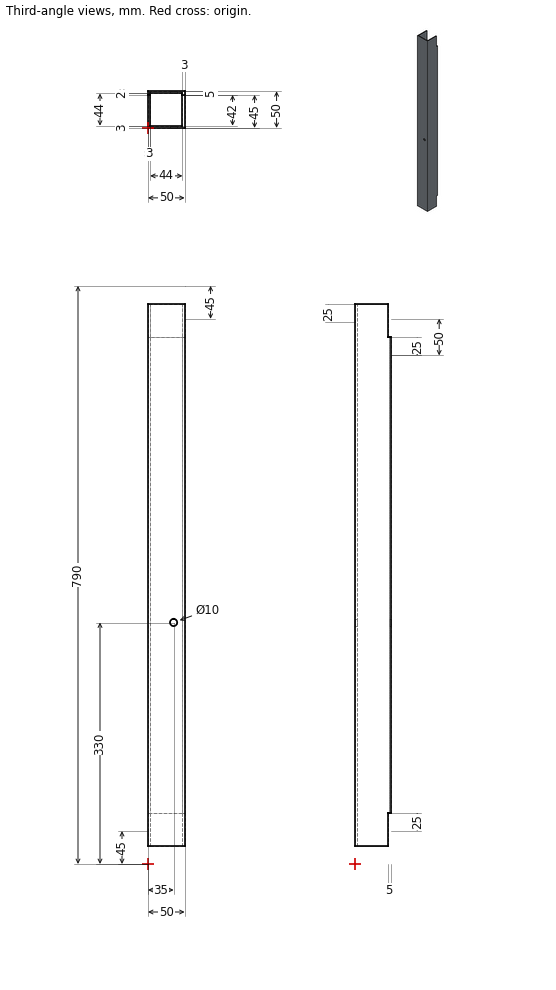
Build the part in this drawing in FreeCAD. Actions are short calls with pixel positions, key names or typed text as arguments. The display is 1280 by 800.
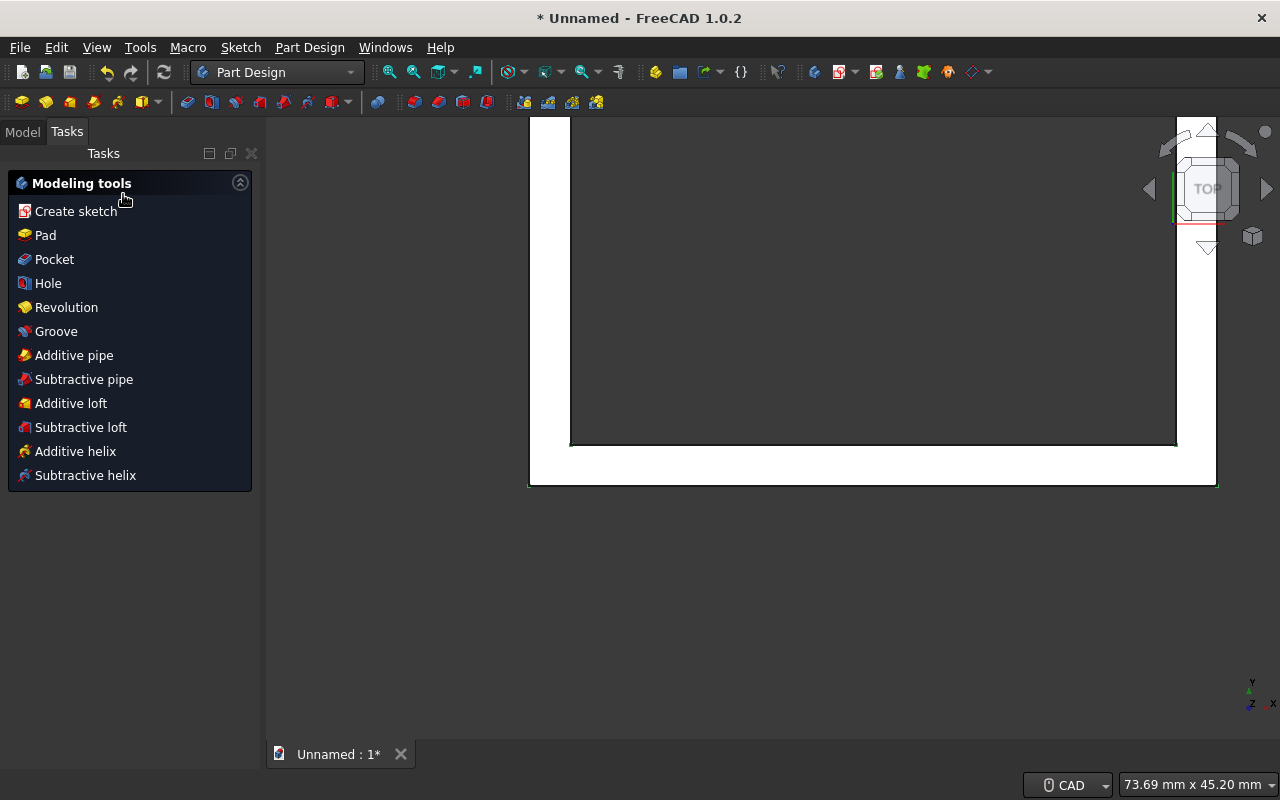
click(22, 102)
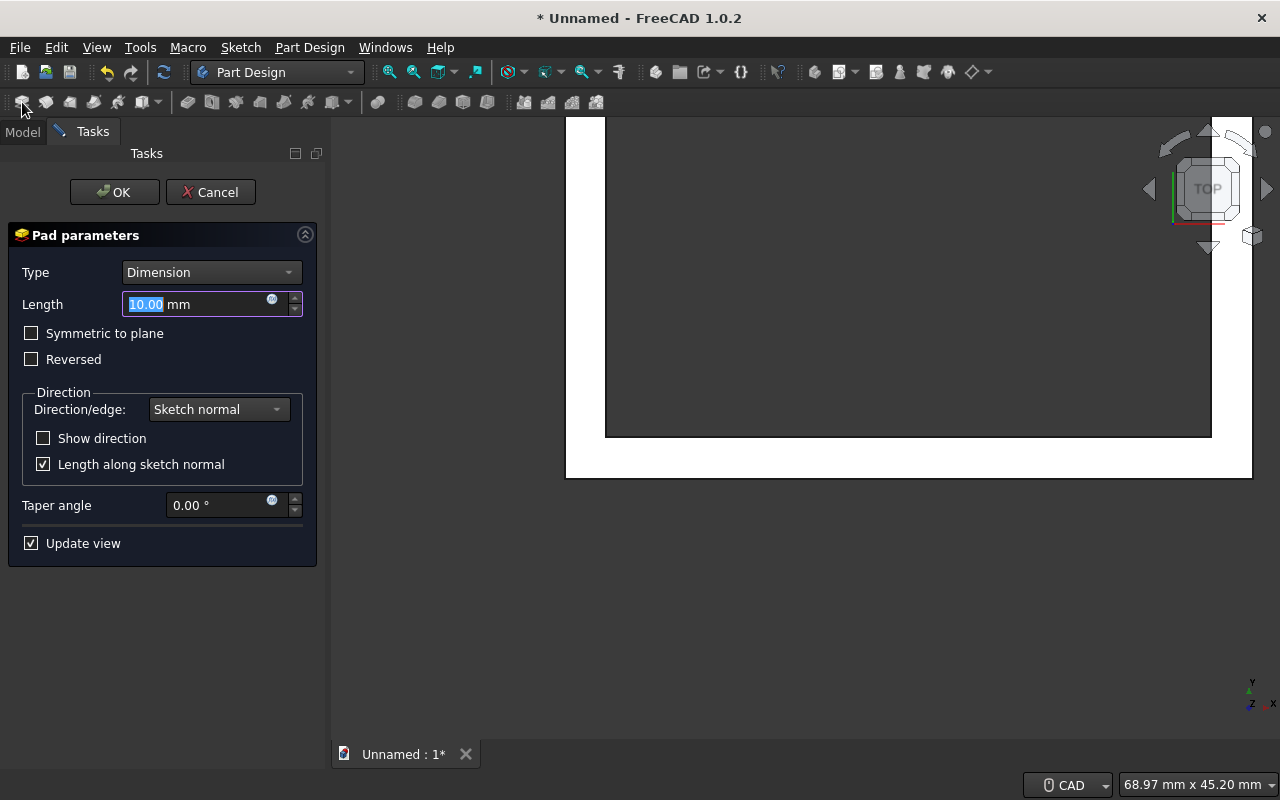
text(25)
key(Tab)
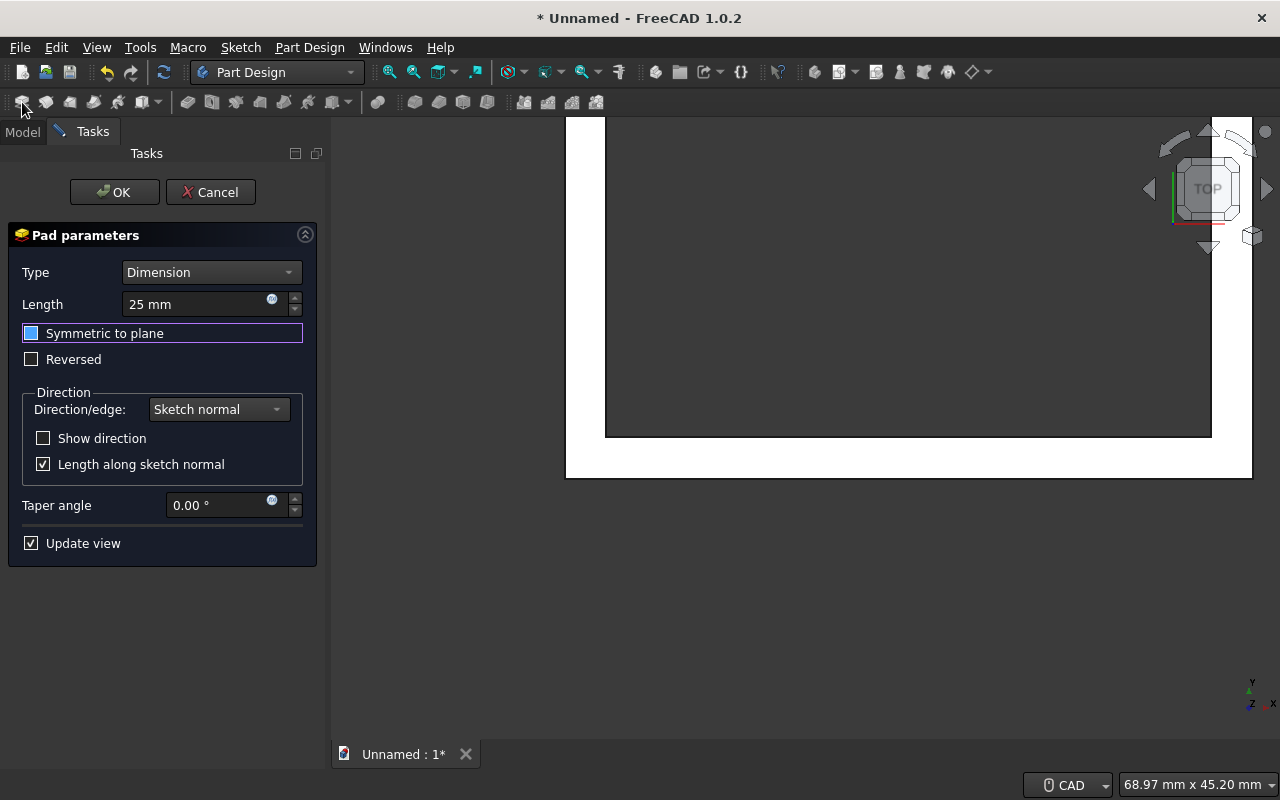
click(115, 192)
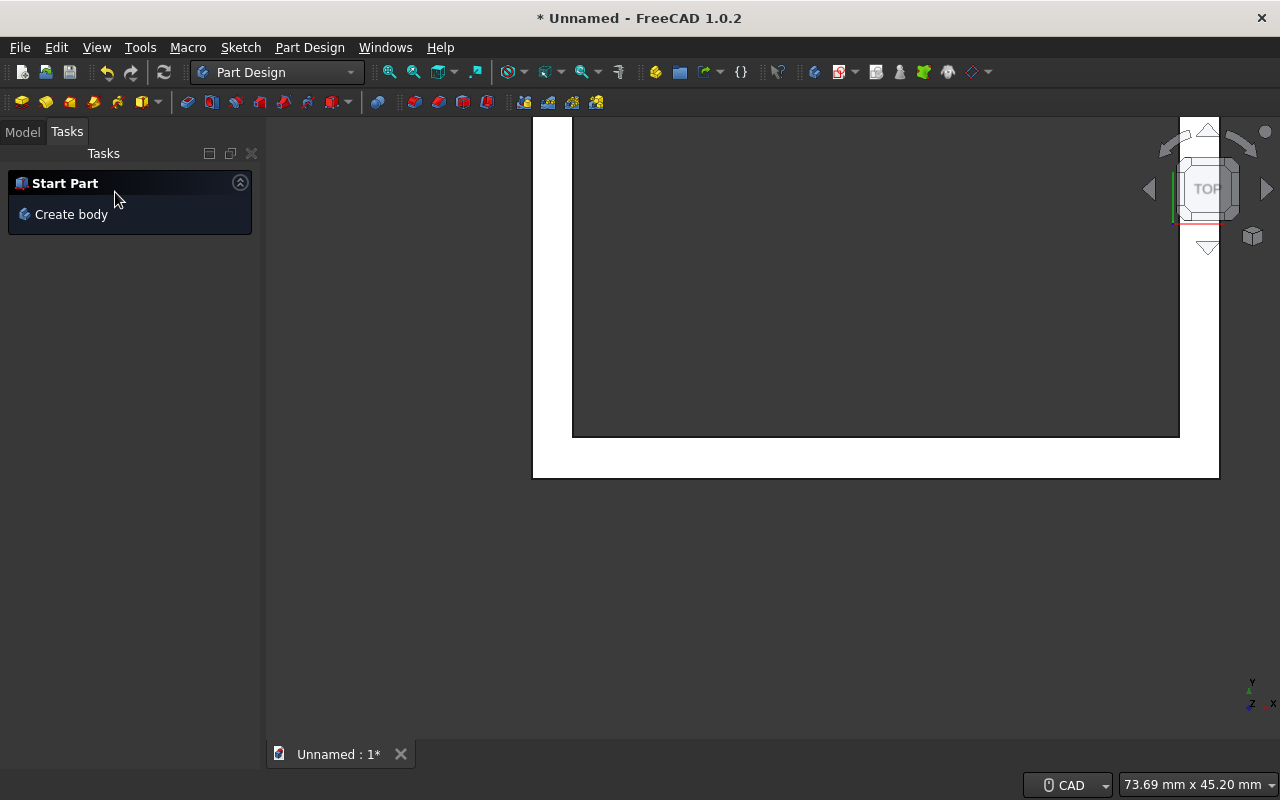
click(390, 72)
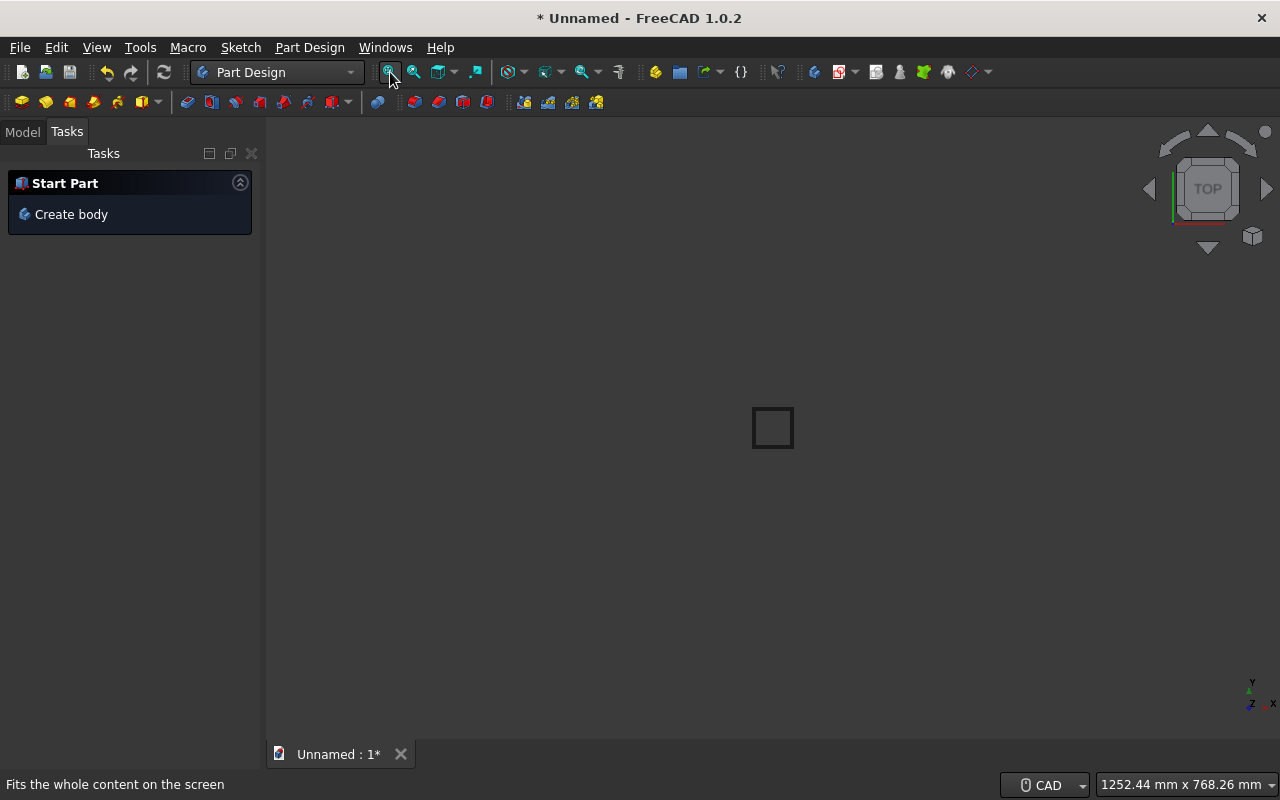
click(840, 72)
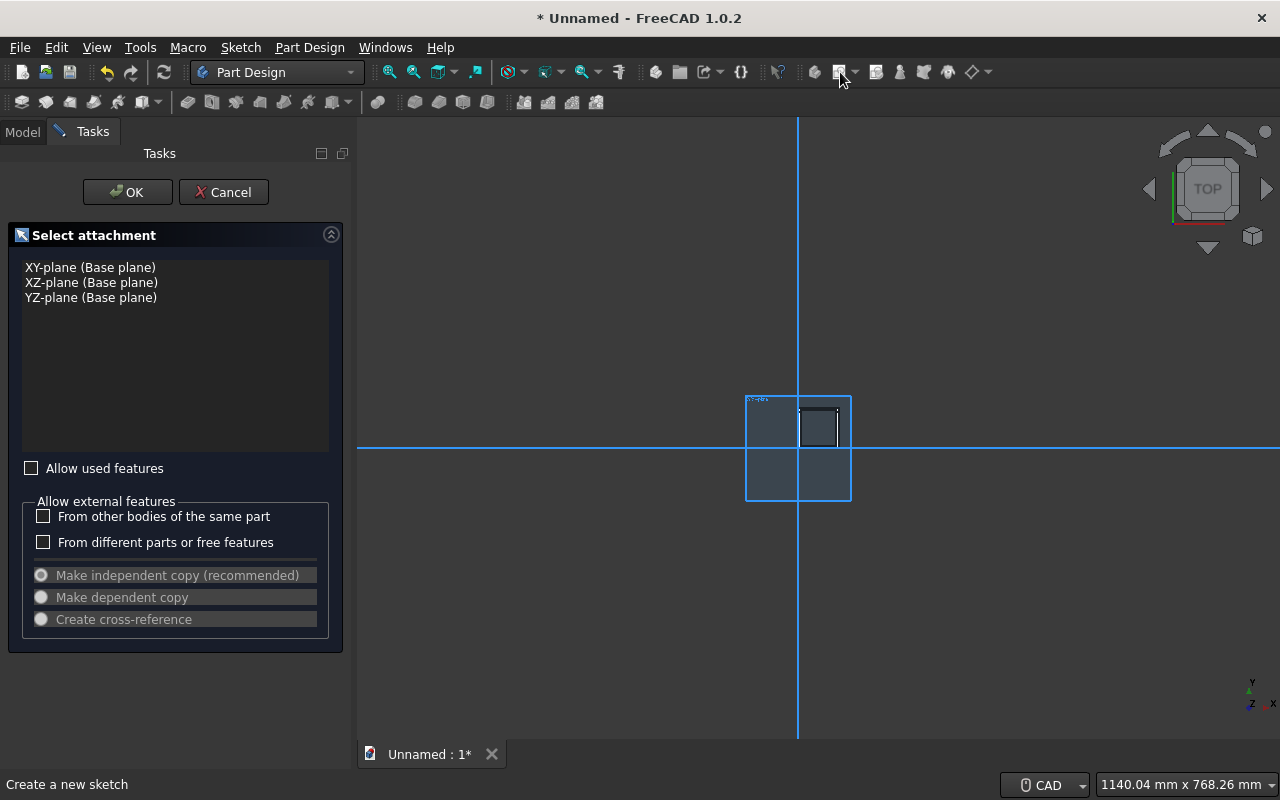
click(82, 268)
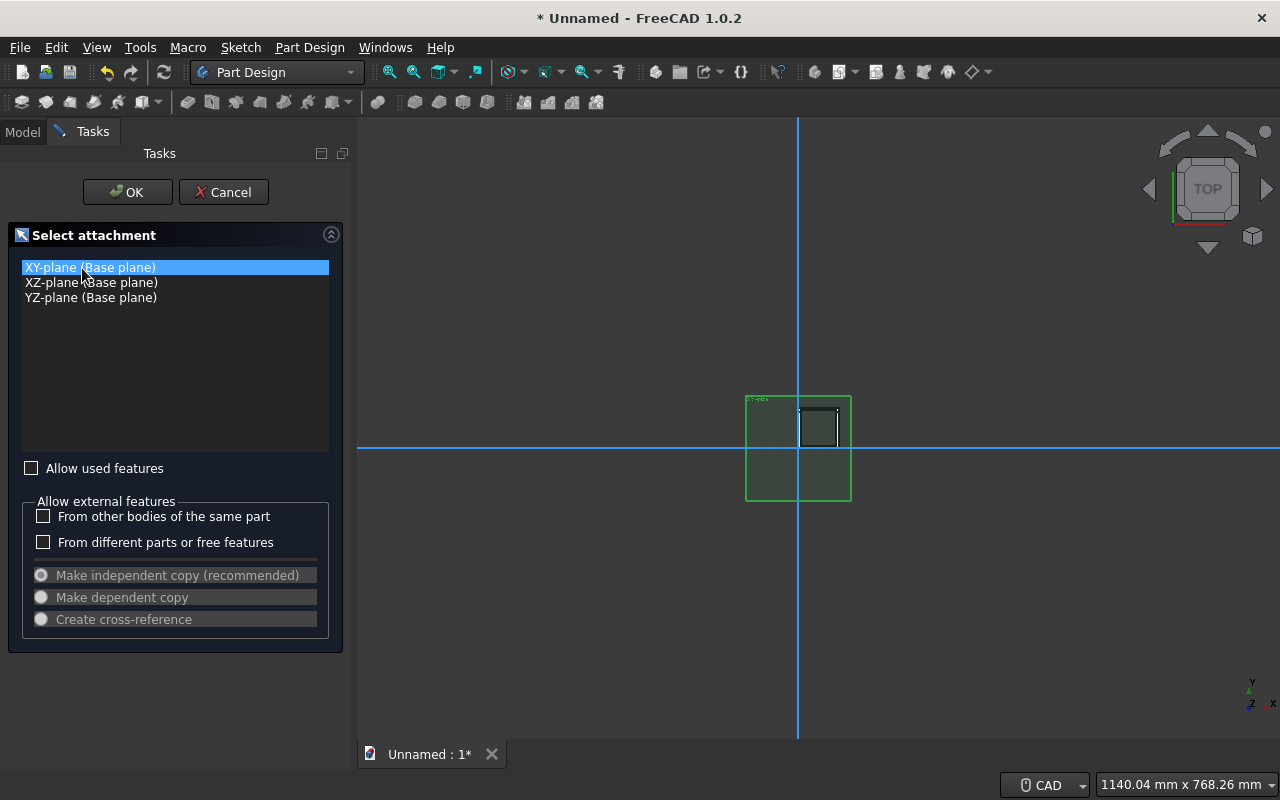
click(128, 192)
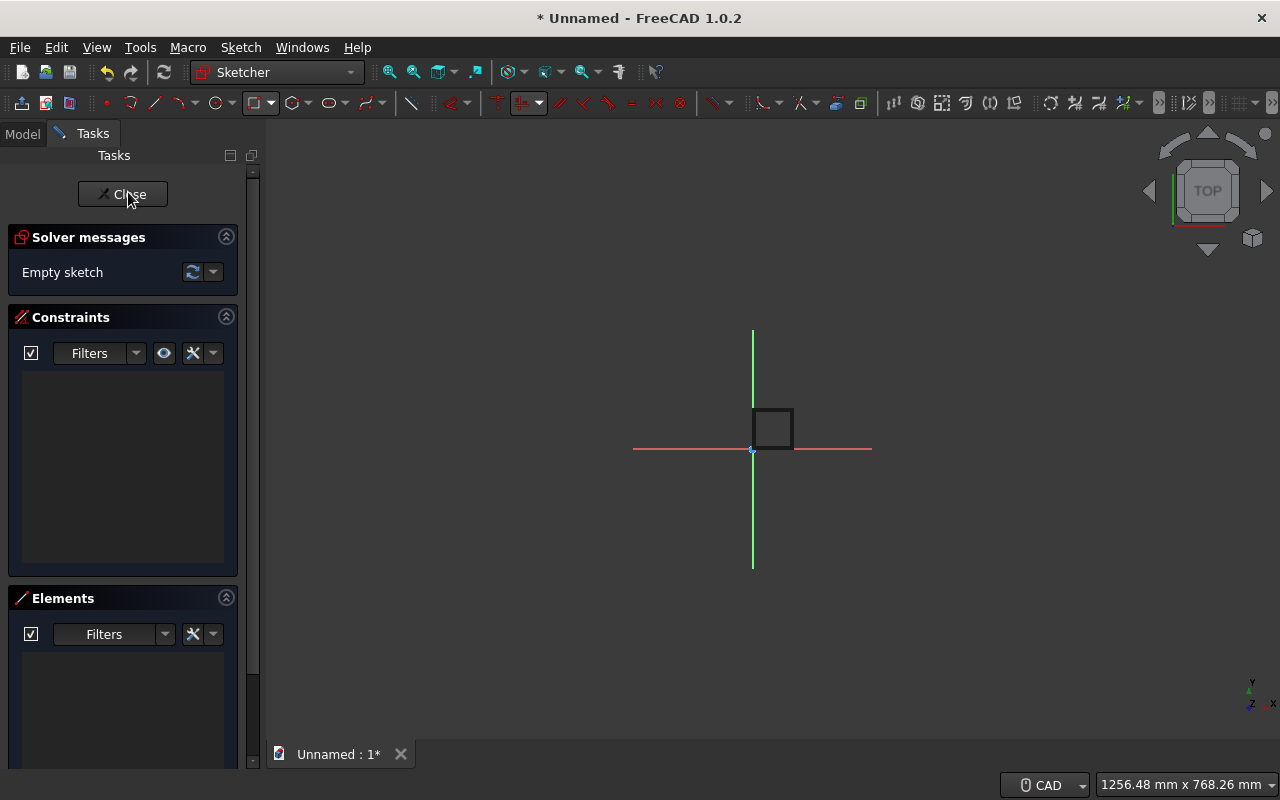
click(70, 104)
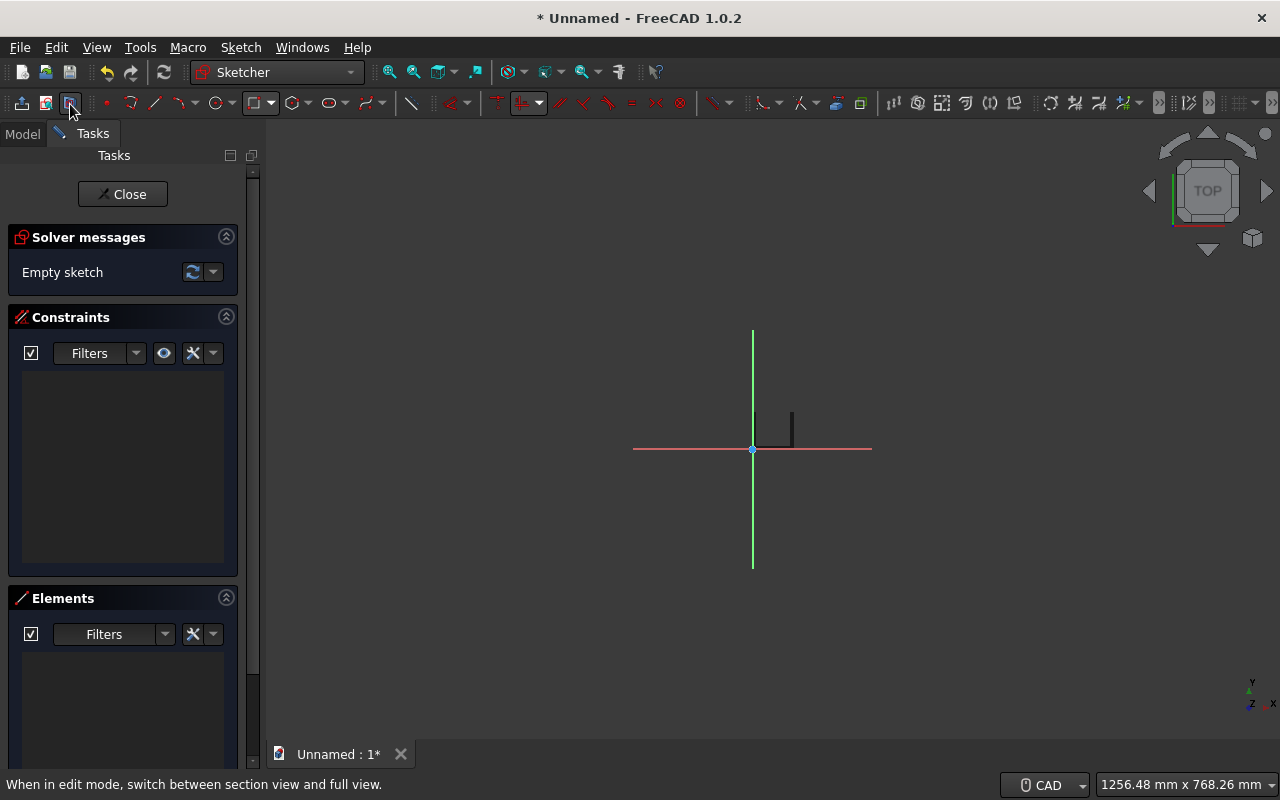
scroll(780, 431, up, 12)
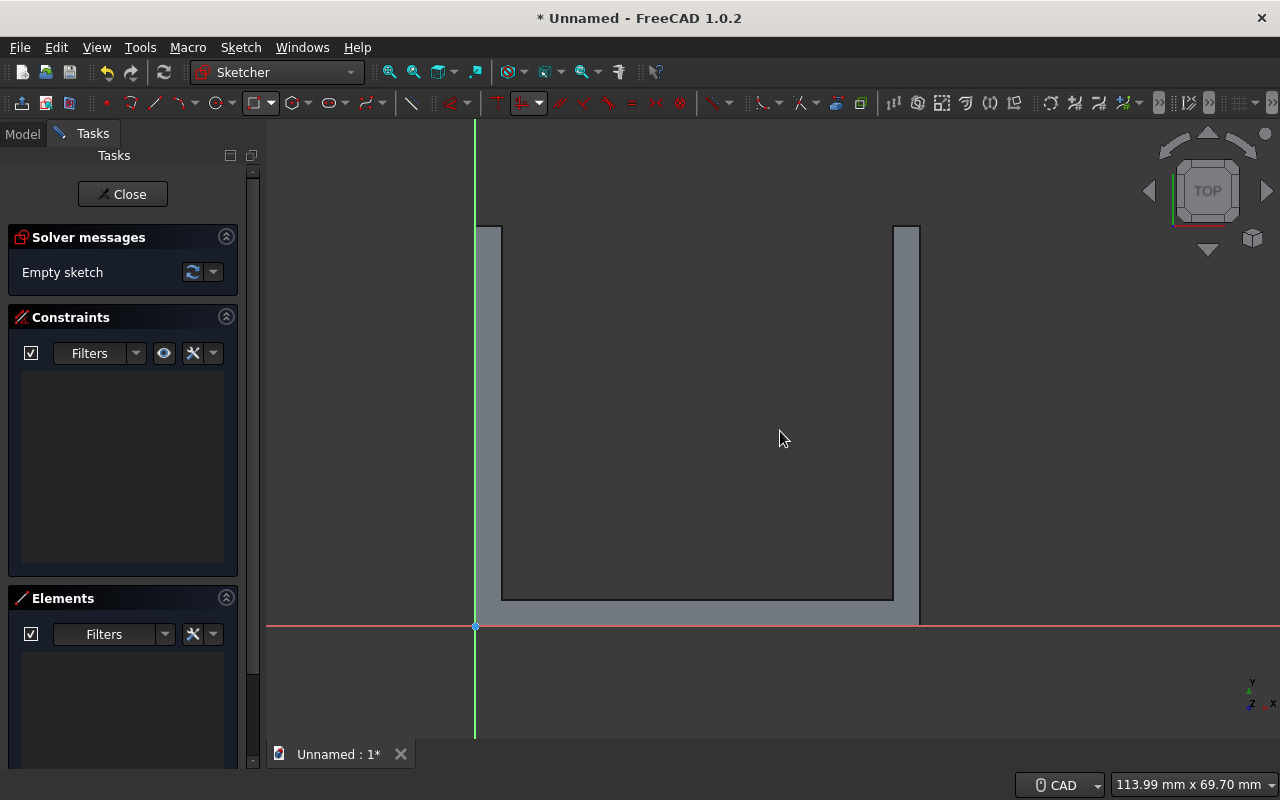
click(132, 104)